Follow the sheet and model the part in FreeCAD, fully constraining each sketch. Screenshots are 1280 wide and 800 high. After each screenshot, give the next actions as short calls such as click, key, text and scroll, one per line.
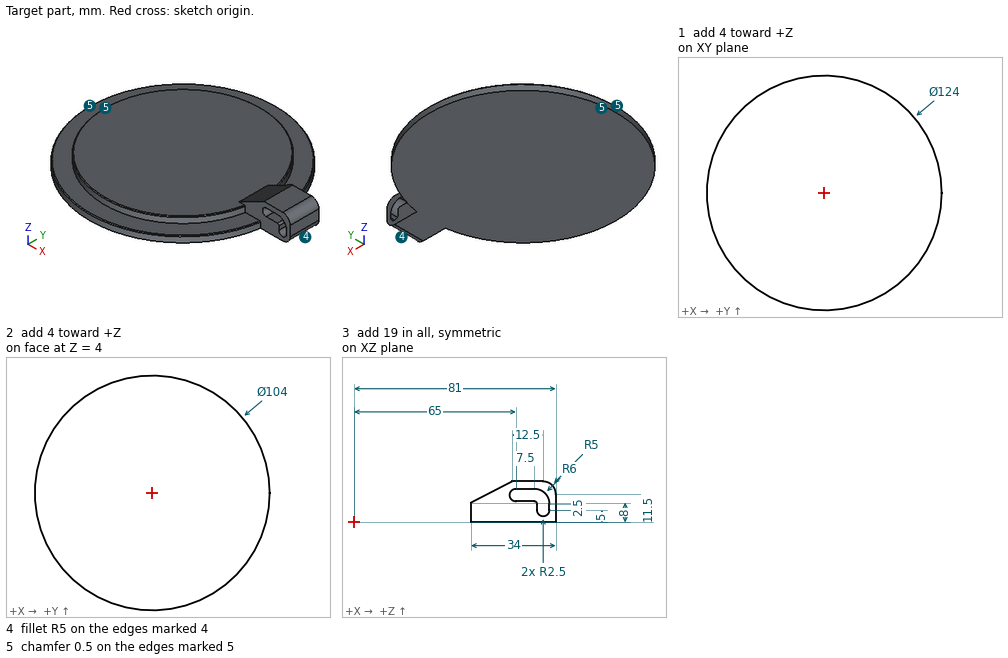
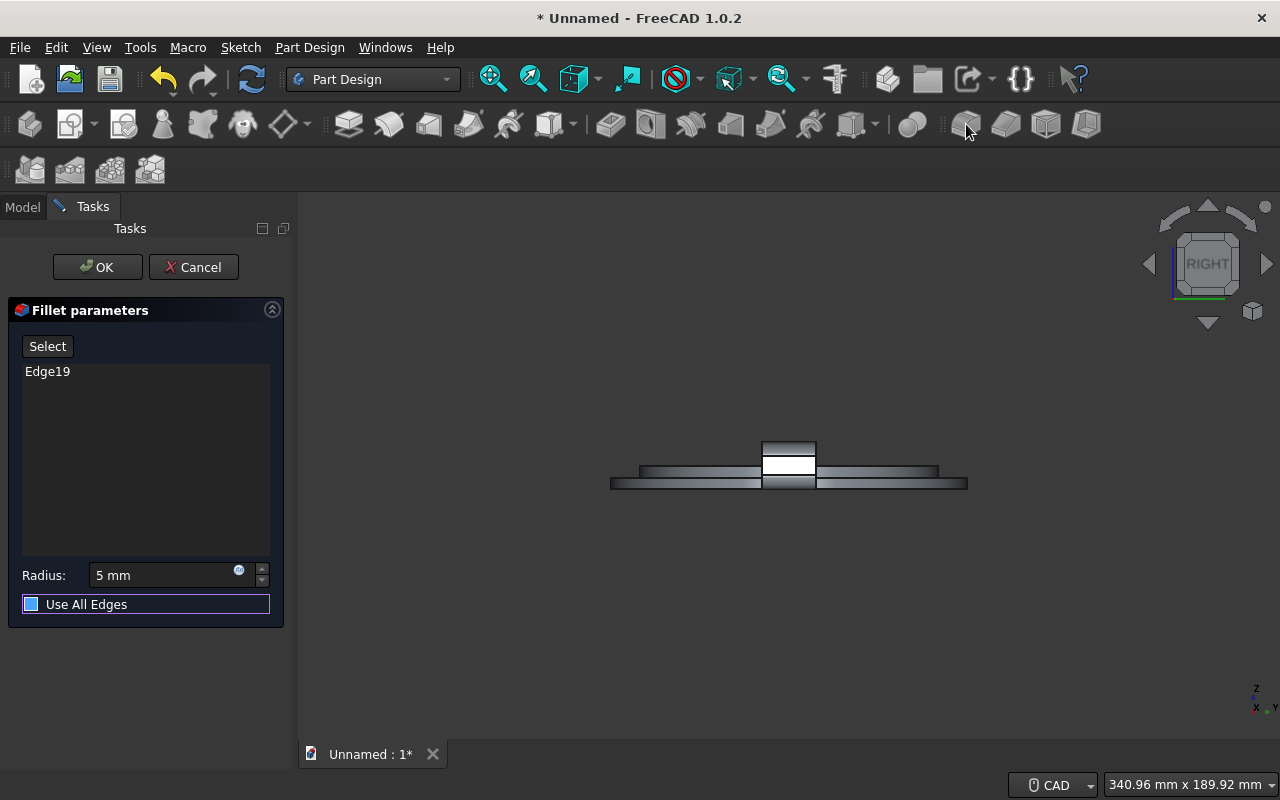
click(98, 267)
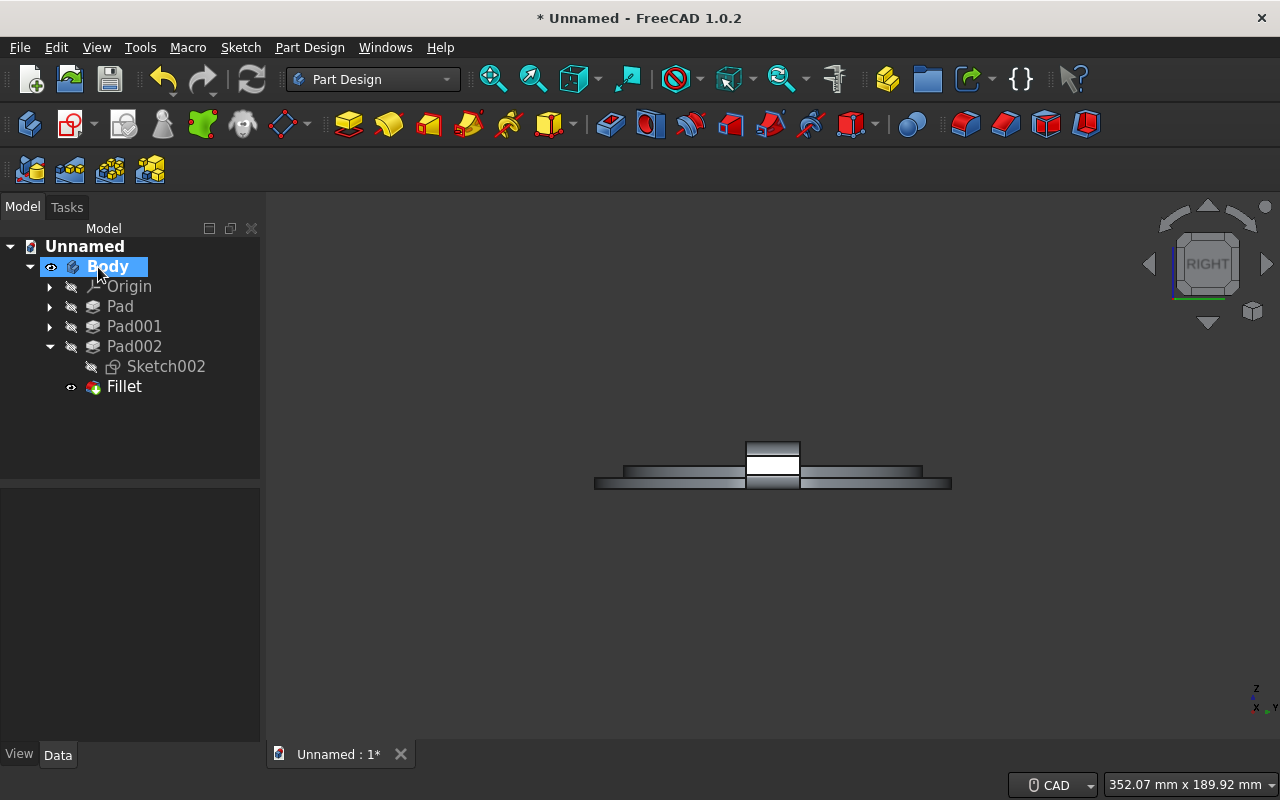
click(494, 80)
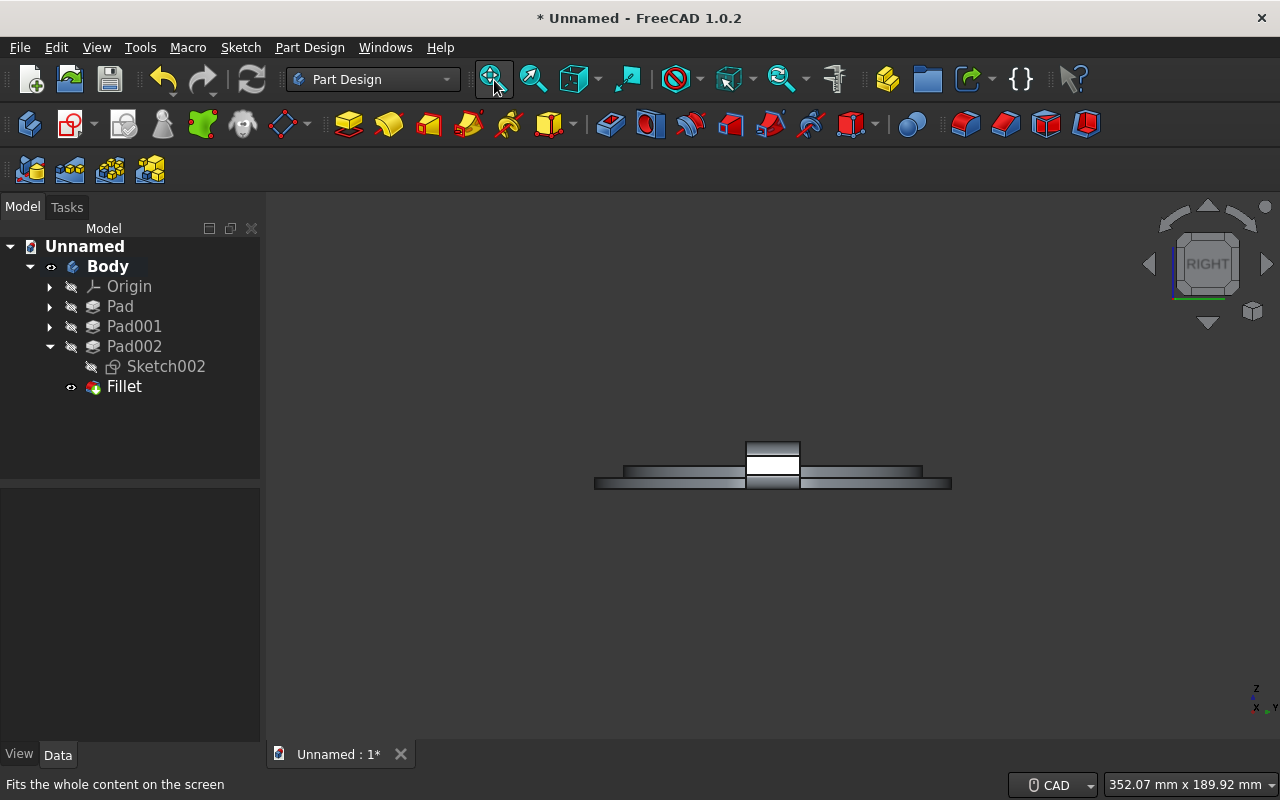
click(873, 477)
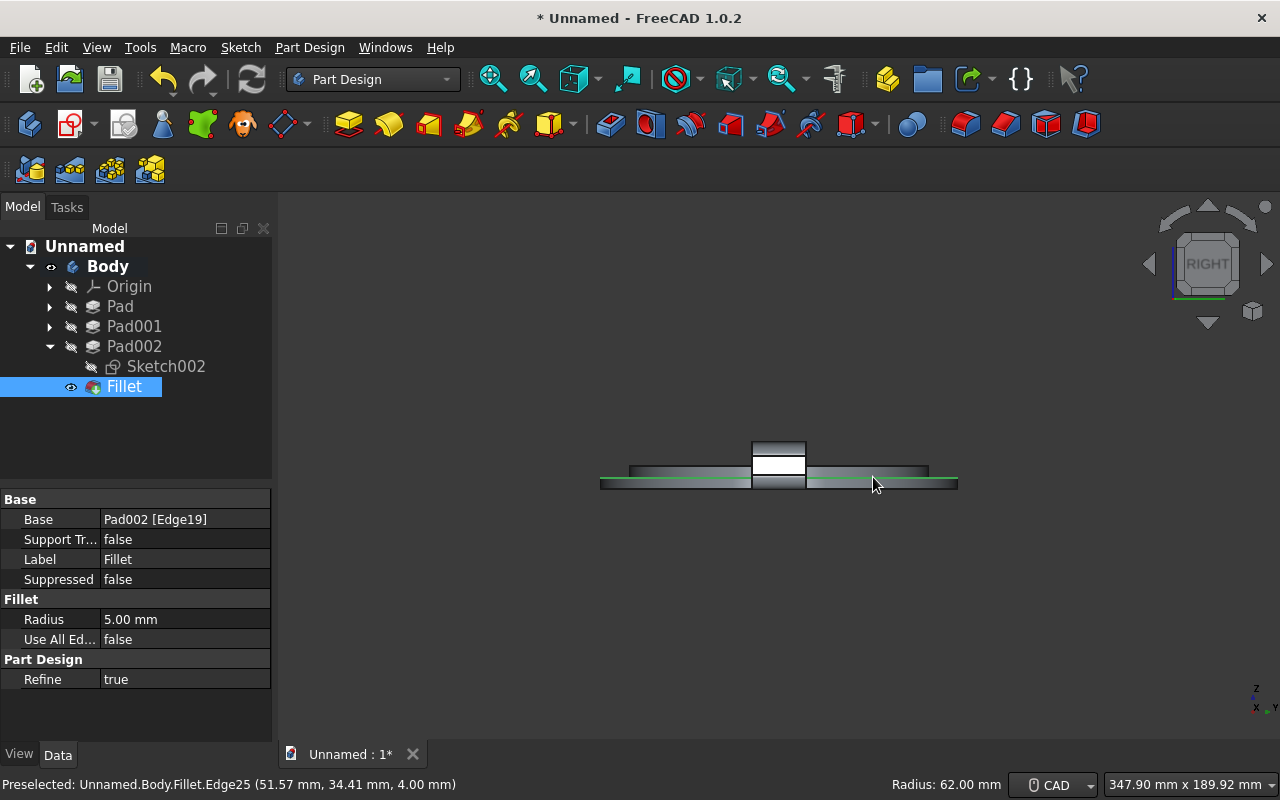
click(863, 465, ctrl)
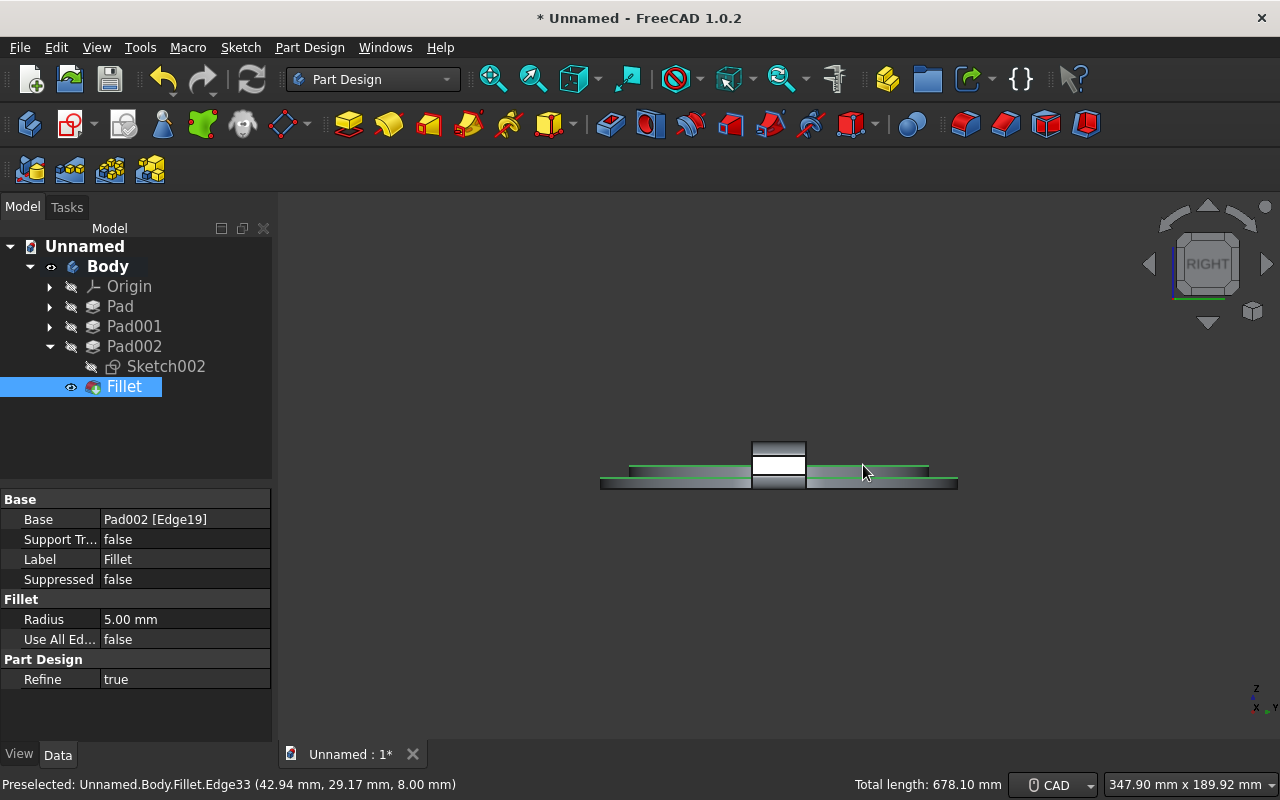
click(1006, 124)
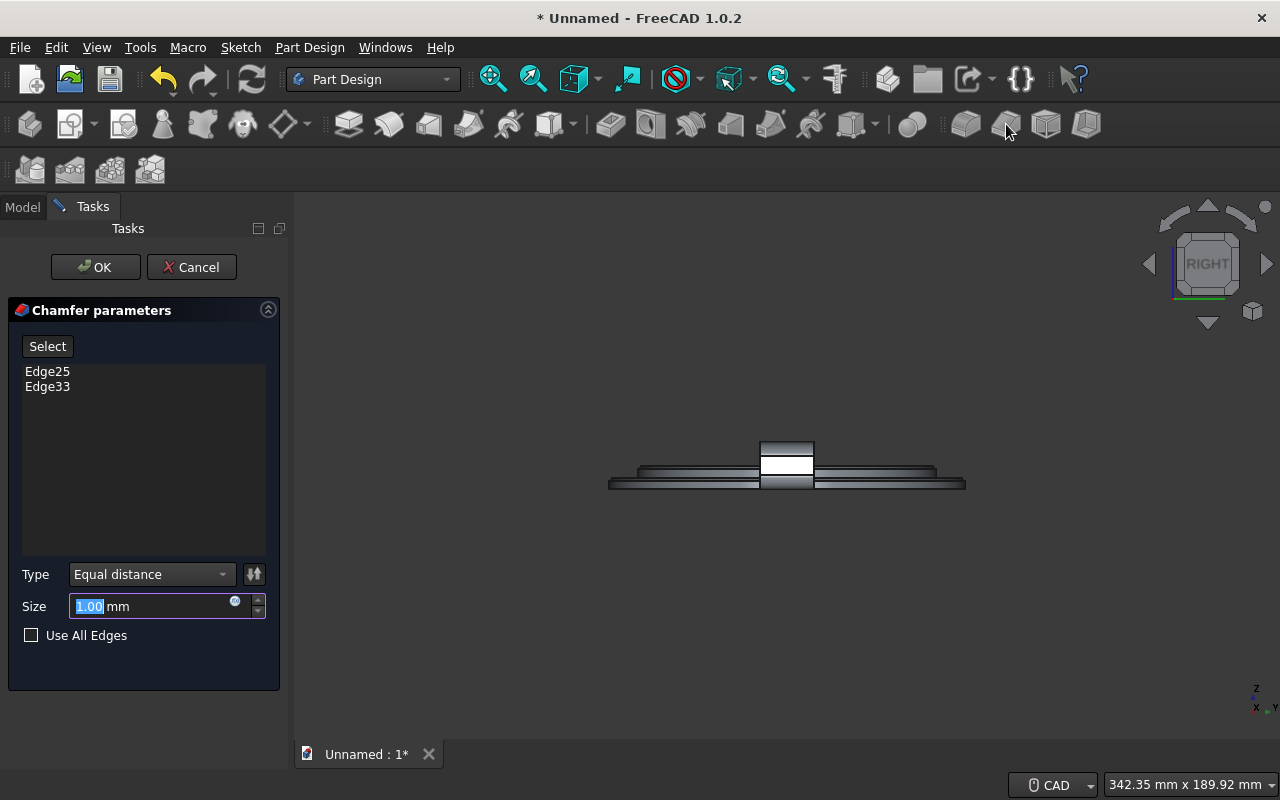
text(0.5)
key(Tab)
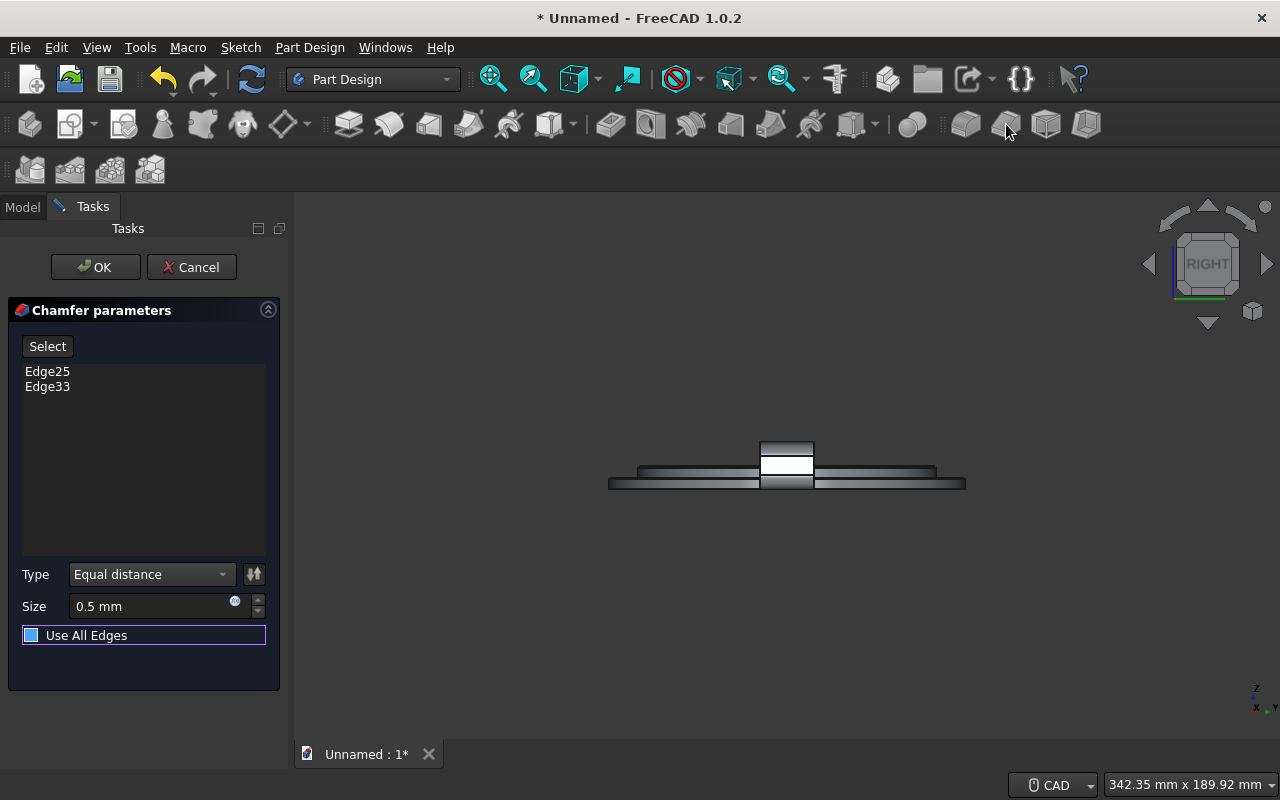
click(96, 267)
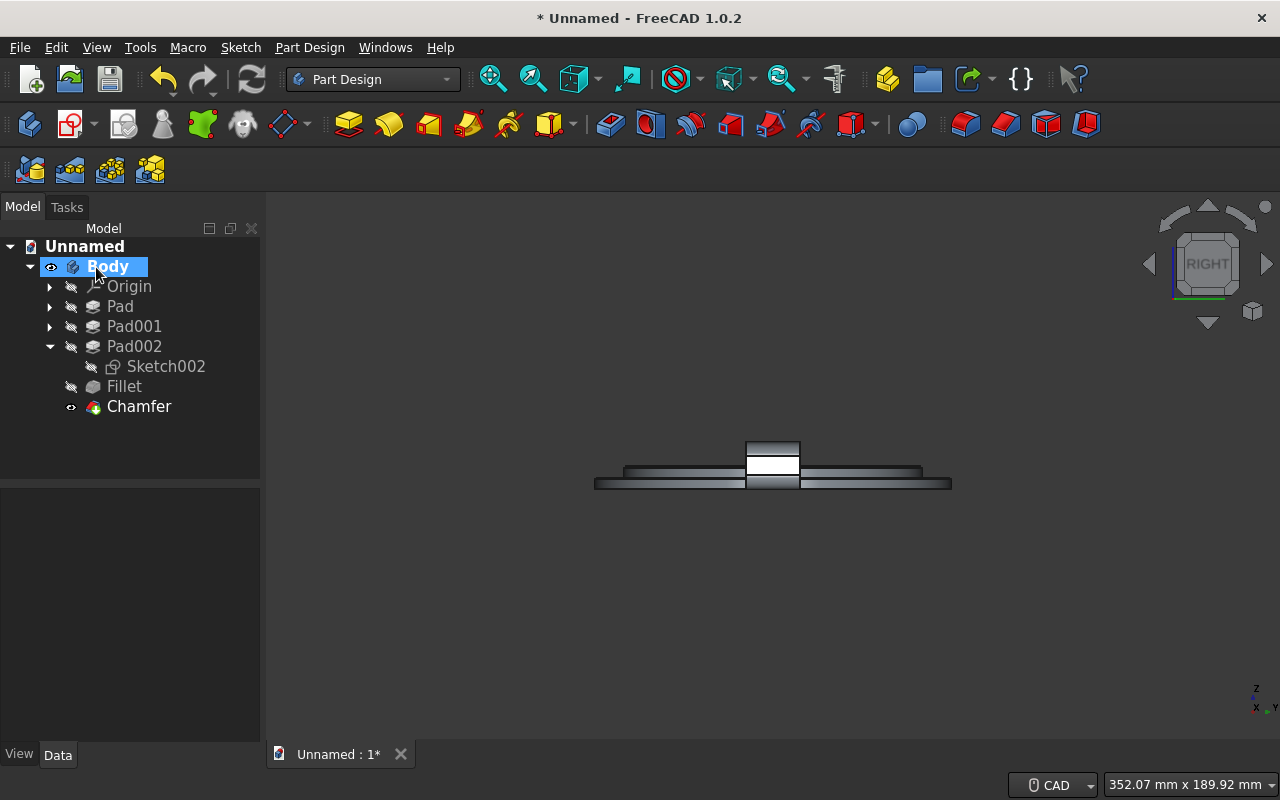
key(0)